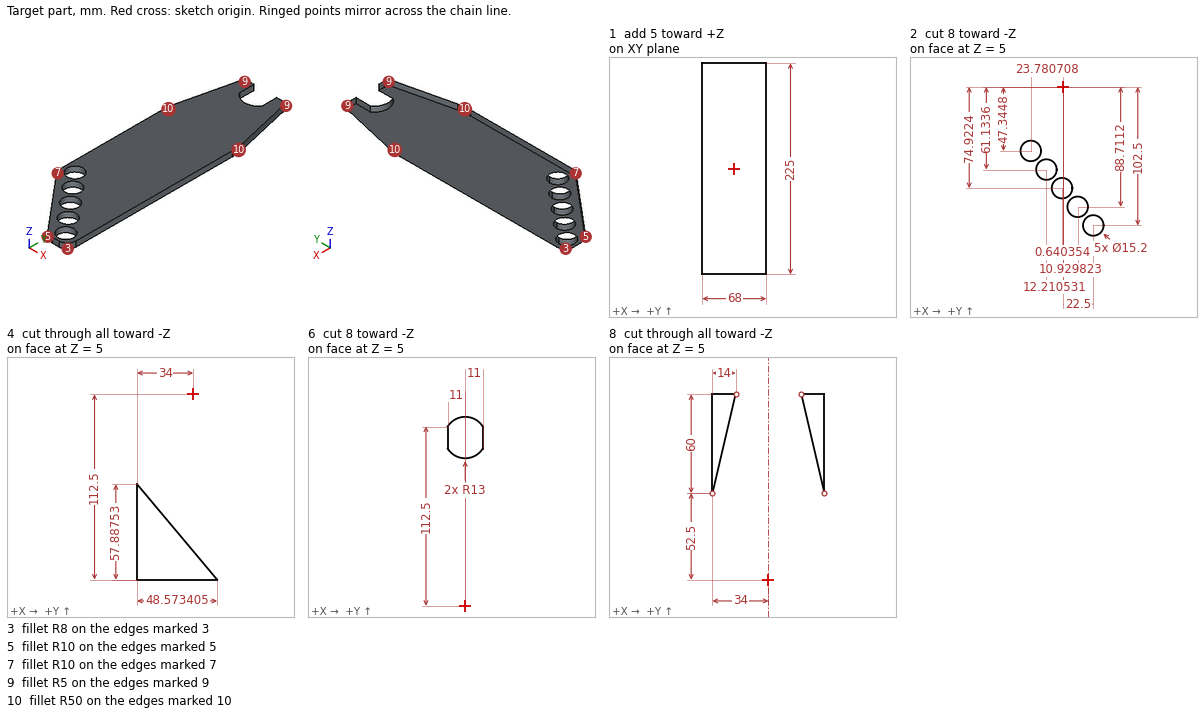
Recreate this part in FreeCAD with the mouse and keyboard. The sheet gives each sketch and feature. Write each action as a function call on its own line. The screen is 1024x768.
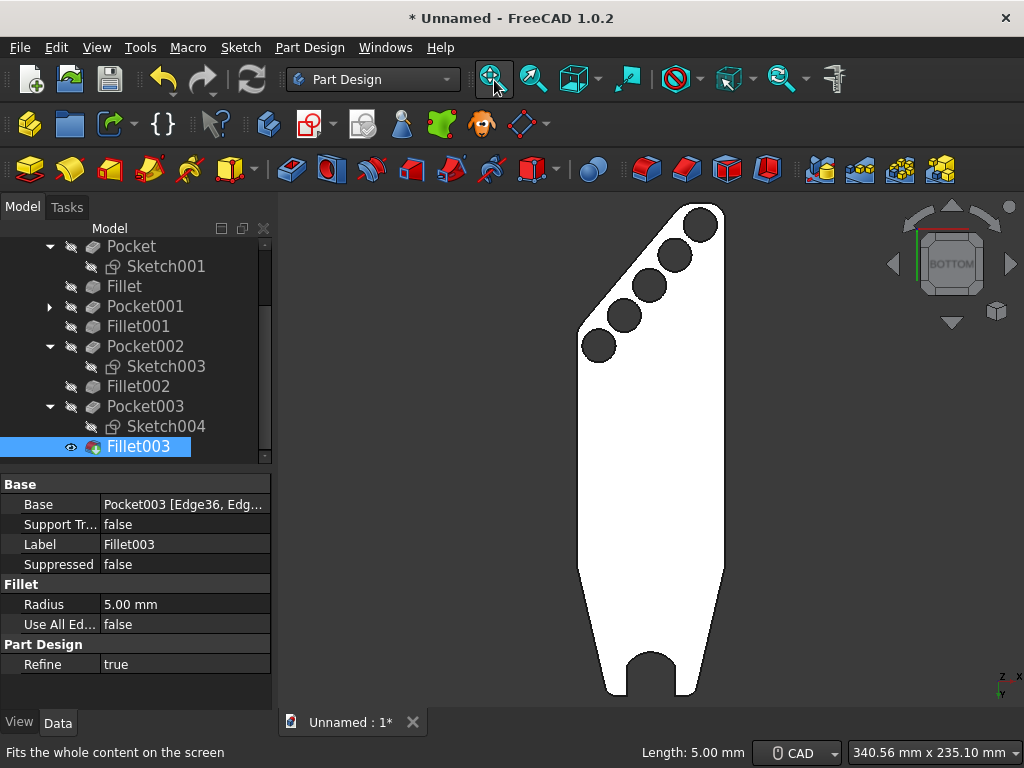
key(4)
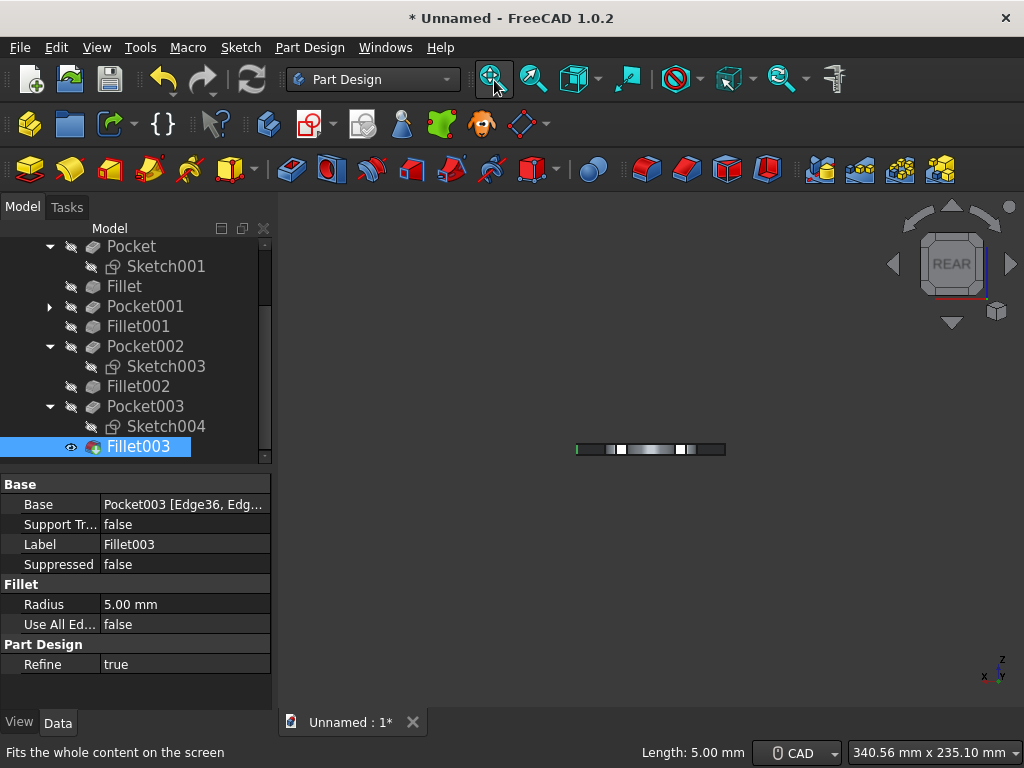
click(494, 80)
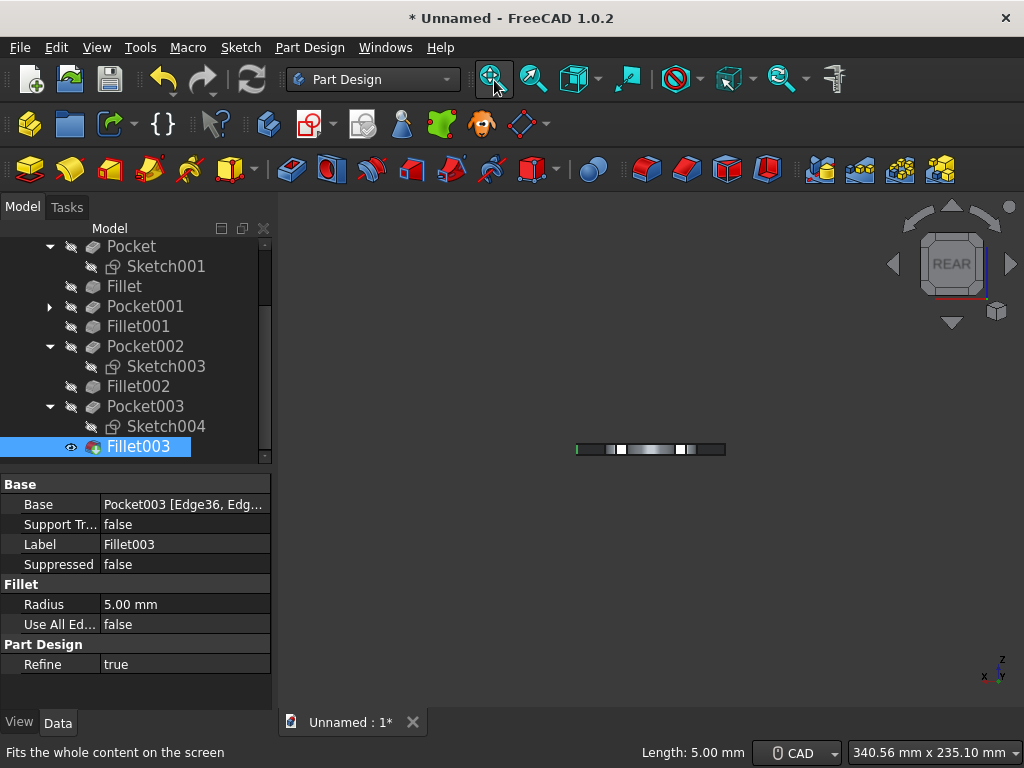
scroll(725, 449, up, 7)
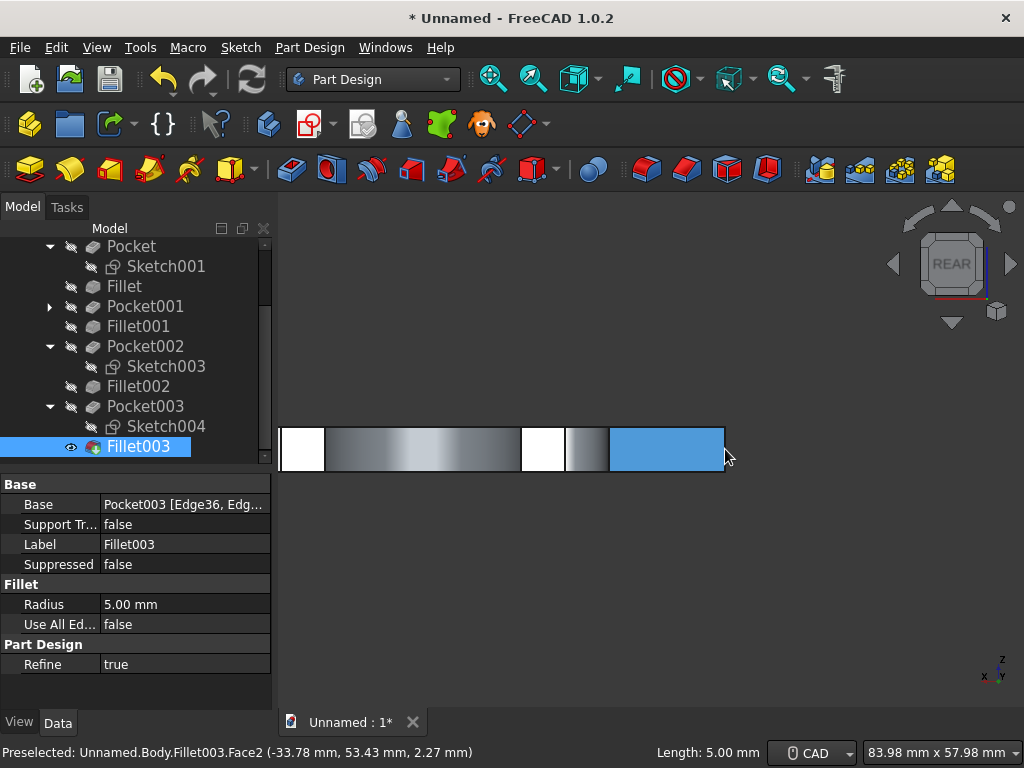
key(v)
key(f)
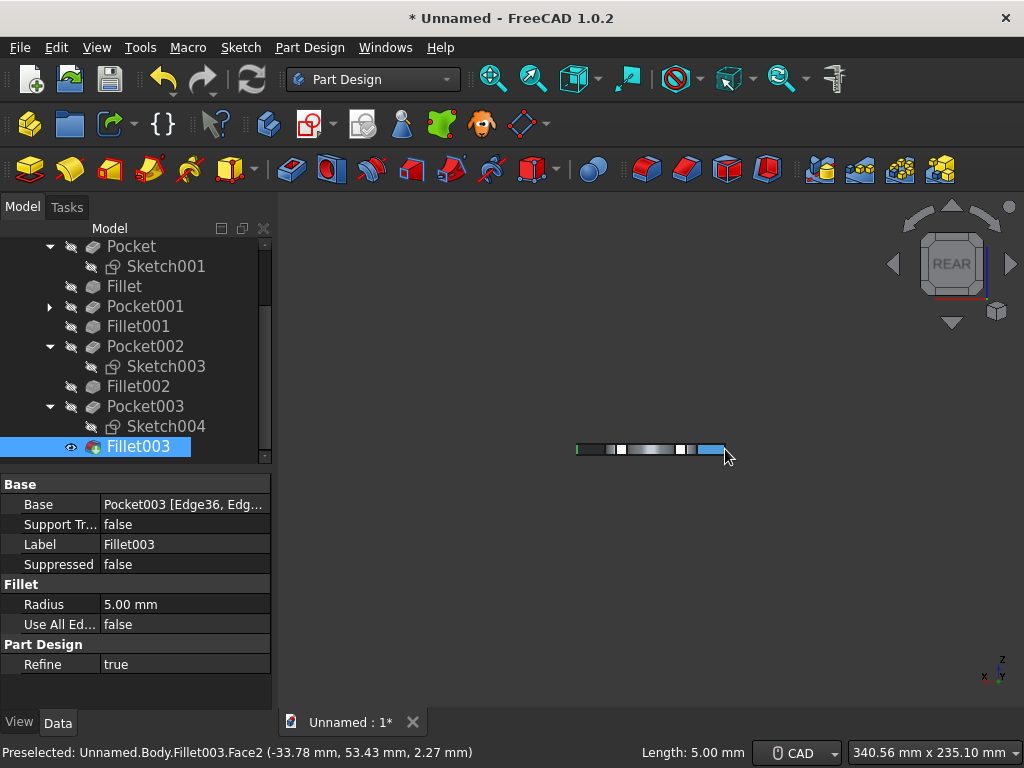
key(6)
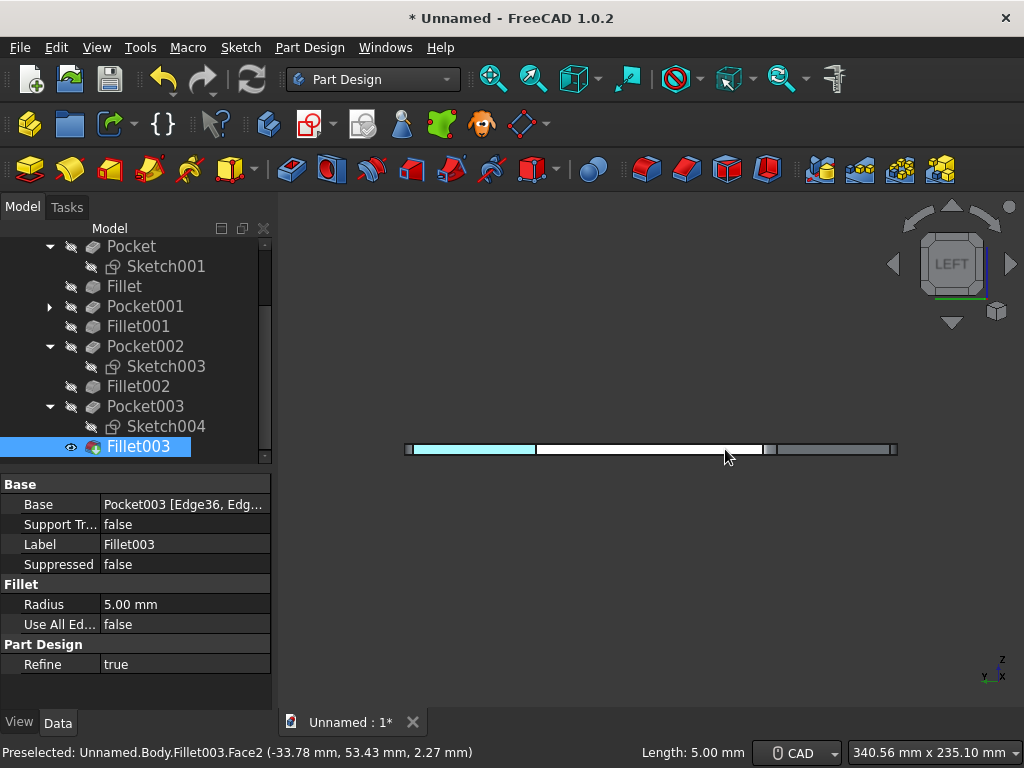
scroll(536, 448, up, 7)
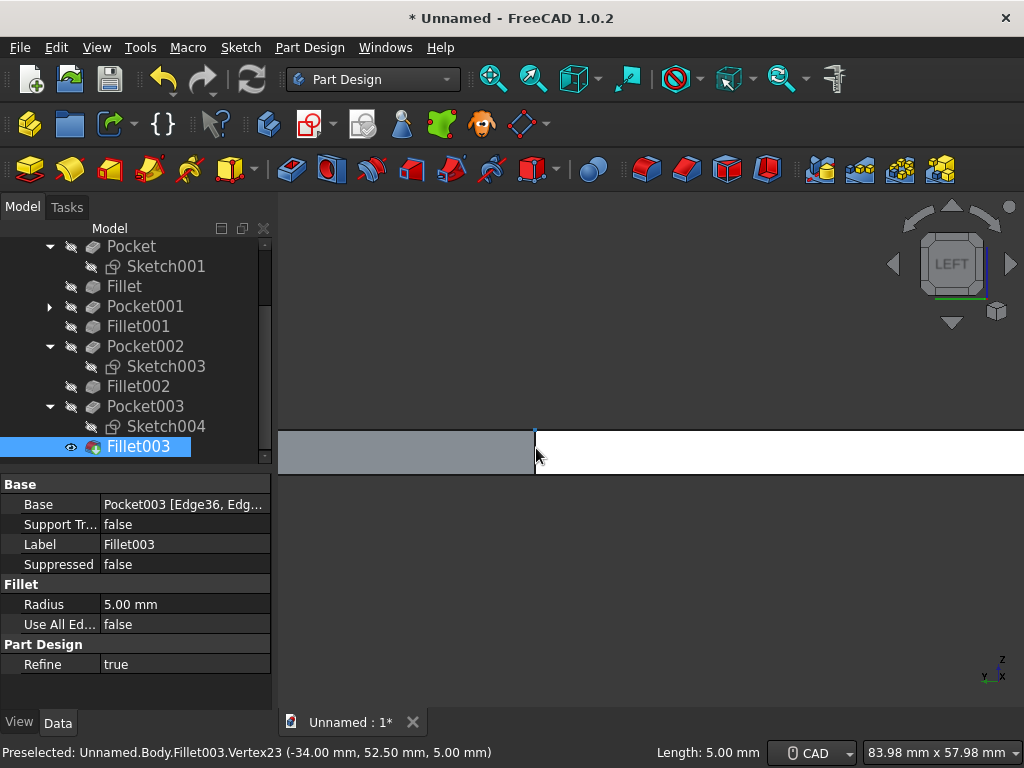
click(535, 452, ctrl)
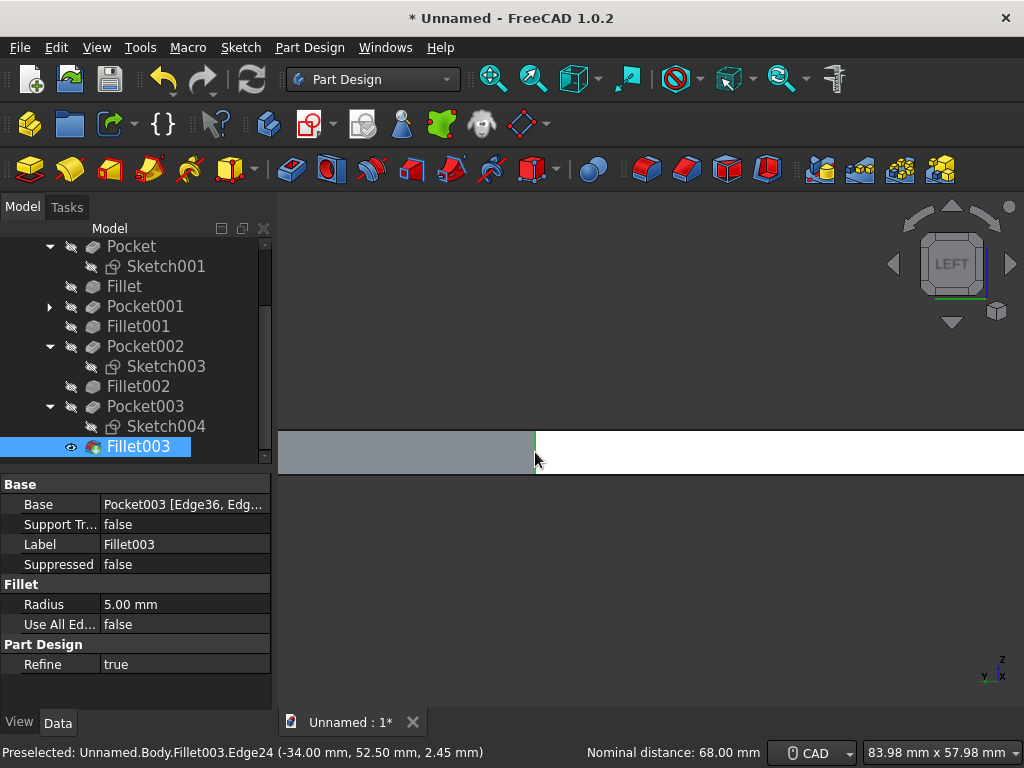
click(648, 170)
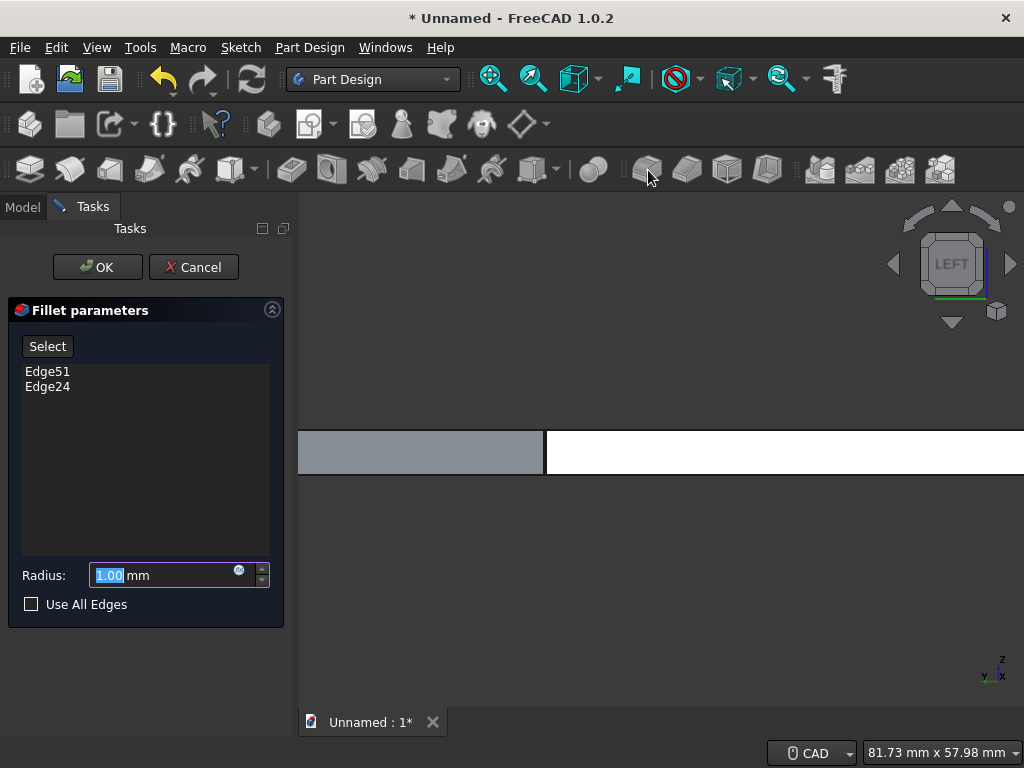
text(50)
key(Tab)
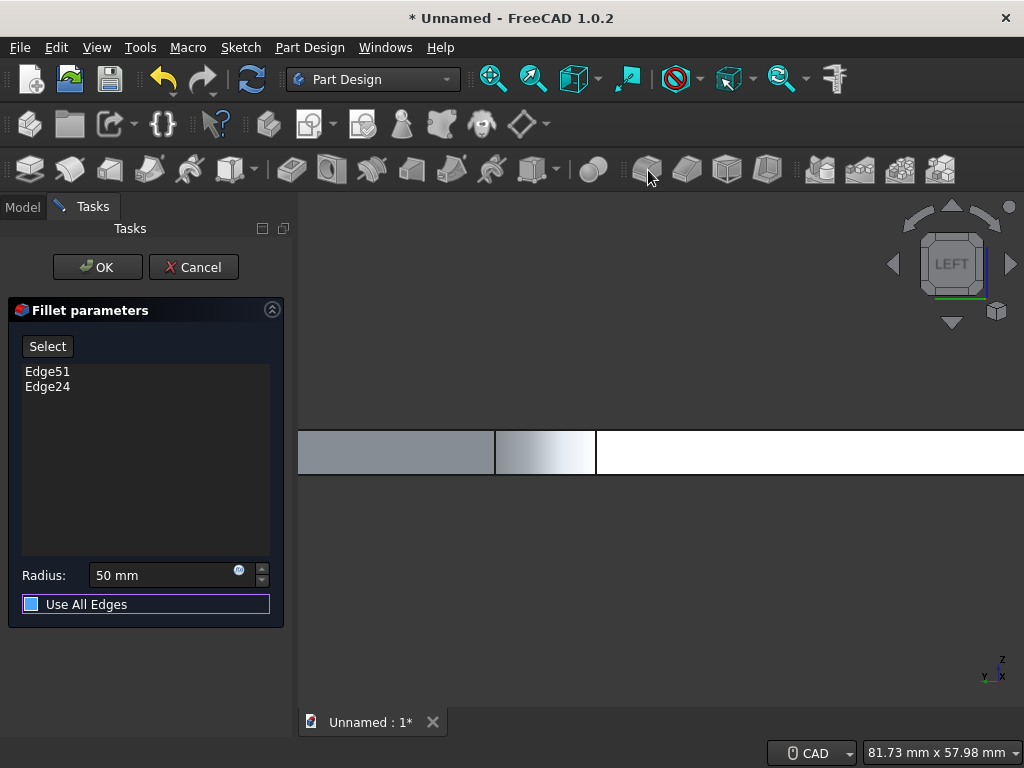
click(98, 267)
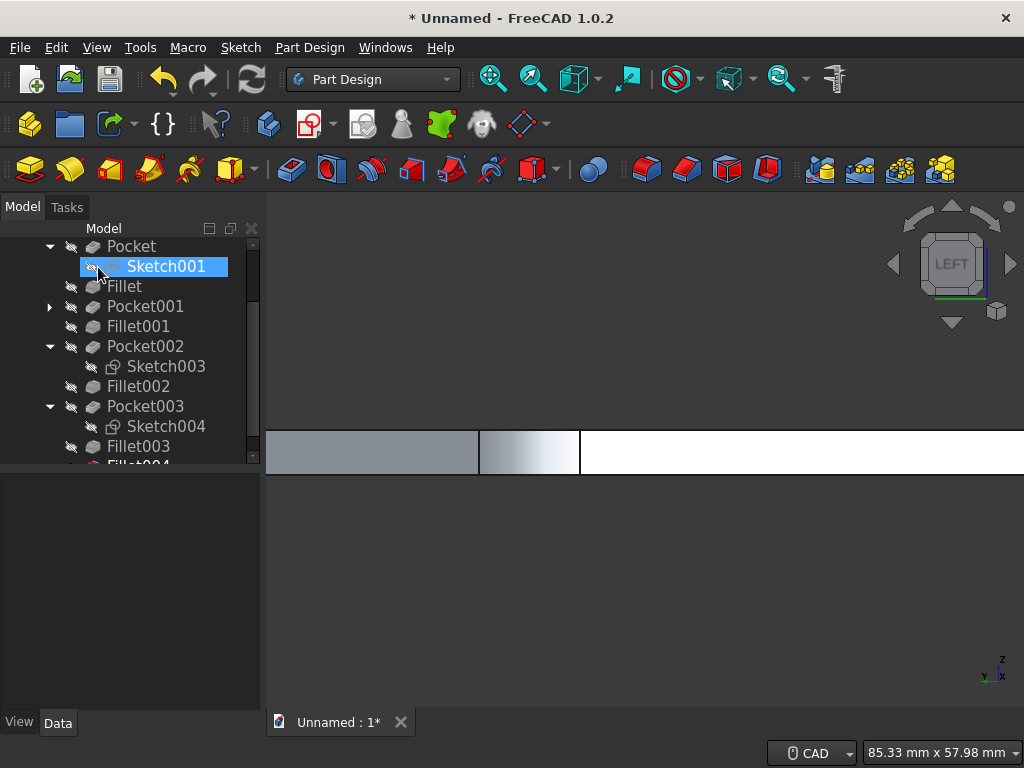
key(0)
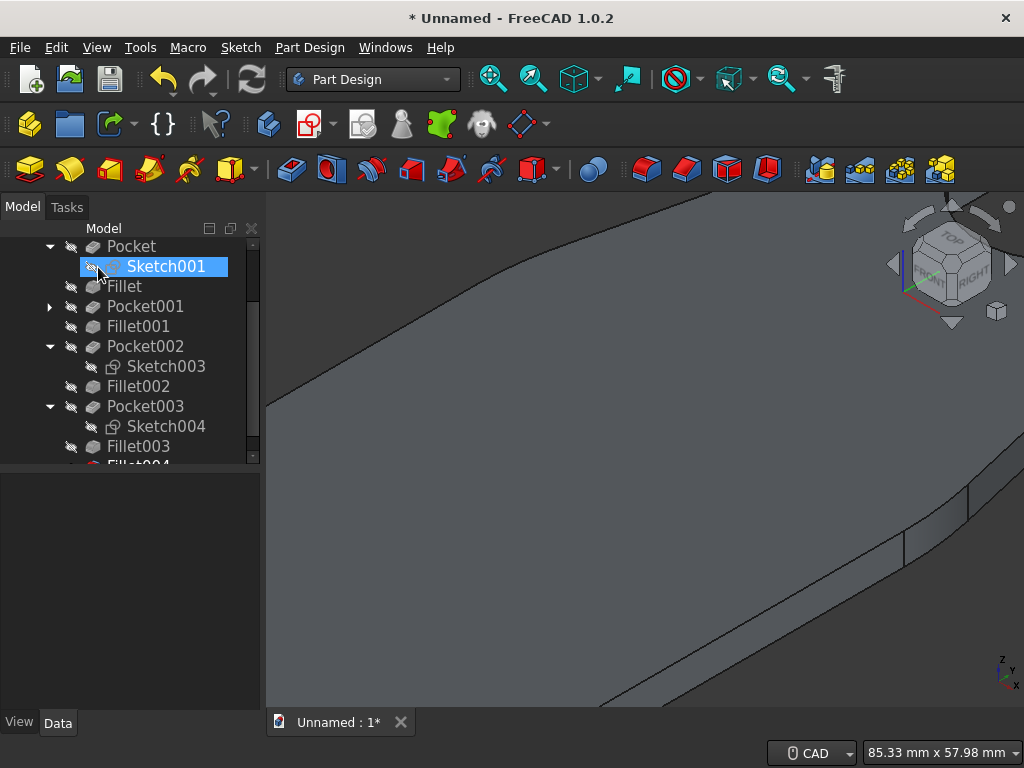
click(494, 80)